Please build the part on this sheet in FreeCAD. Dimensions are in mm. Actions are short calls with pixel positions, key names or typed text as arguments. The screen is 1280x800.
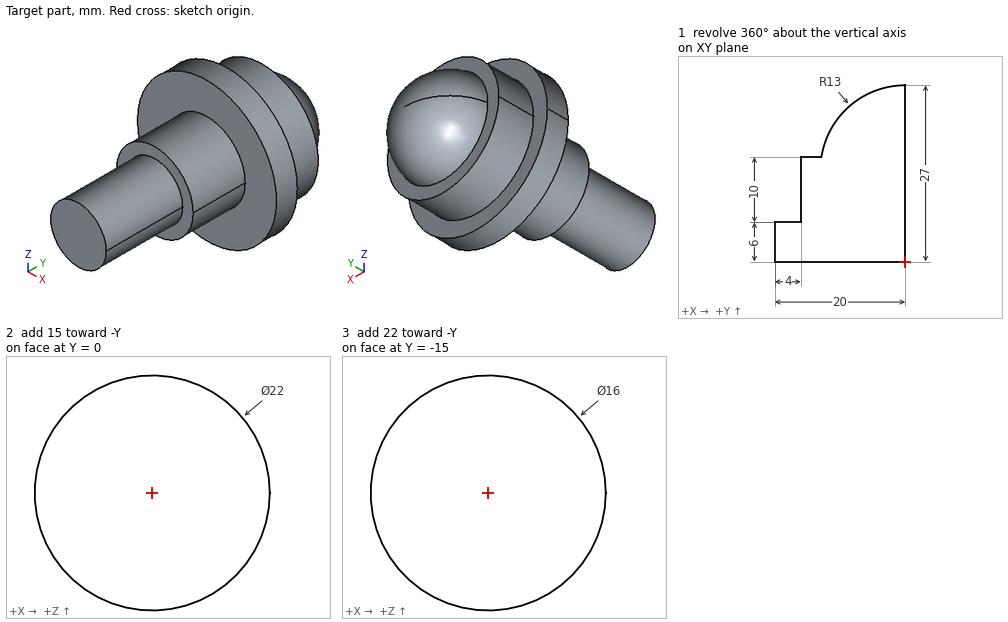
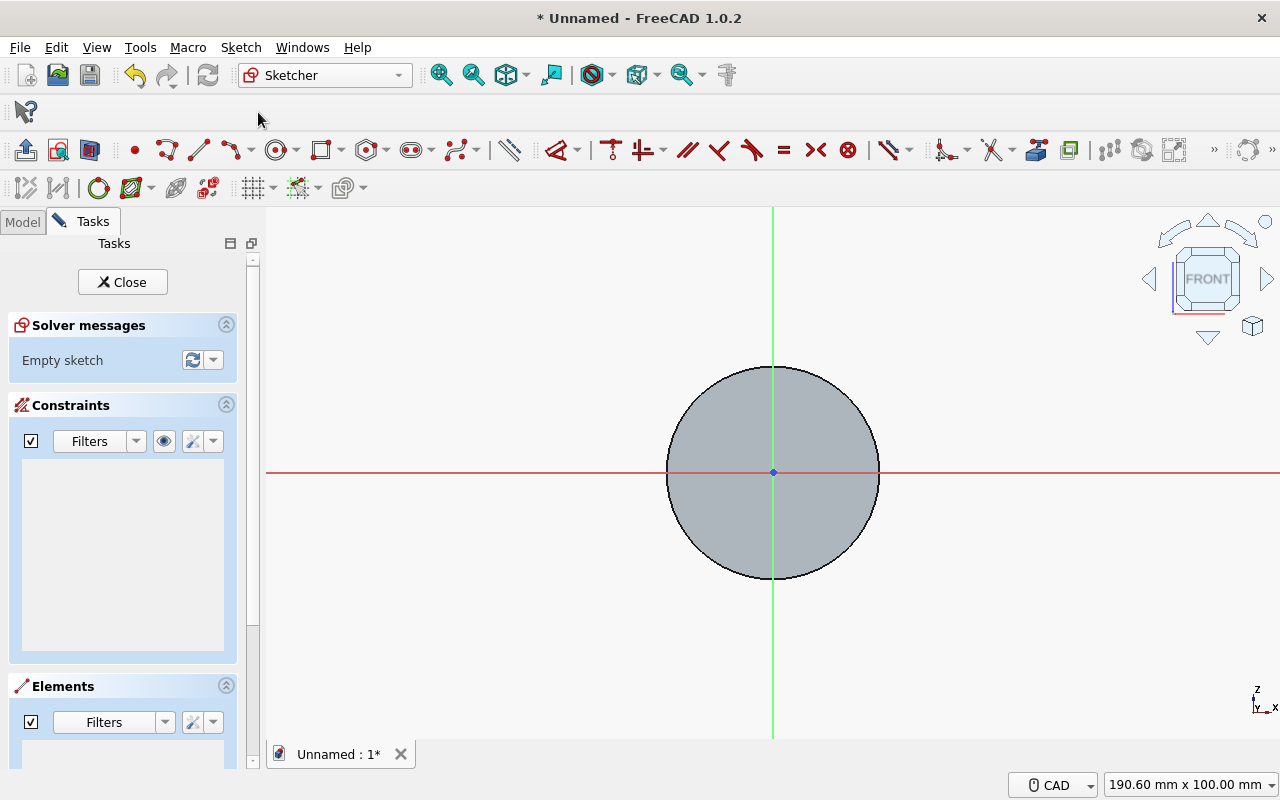
scroll(813, 473, up, 5)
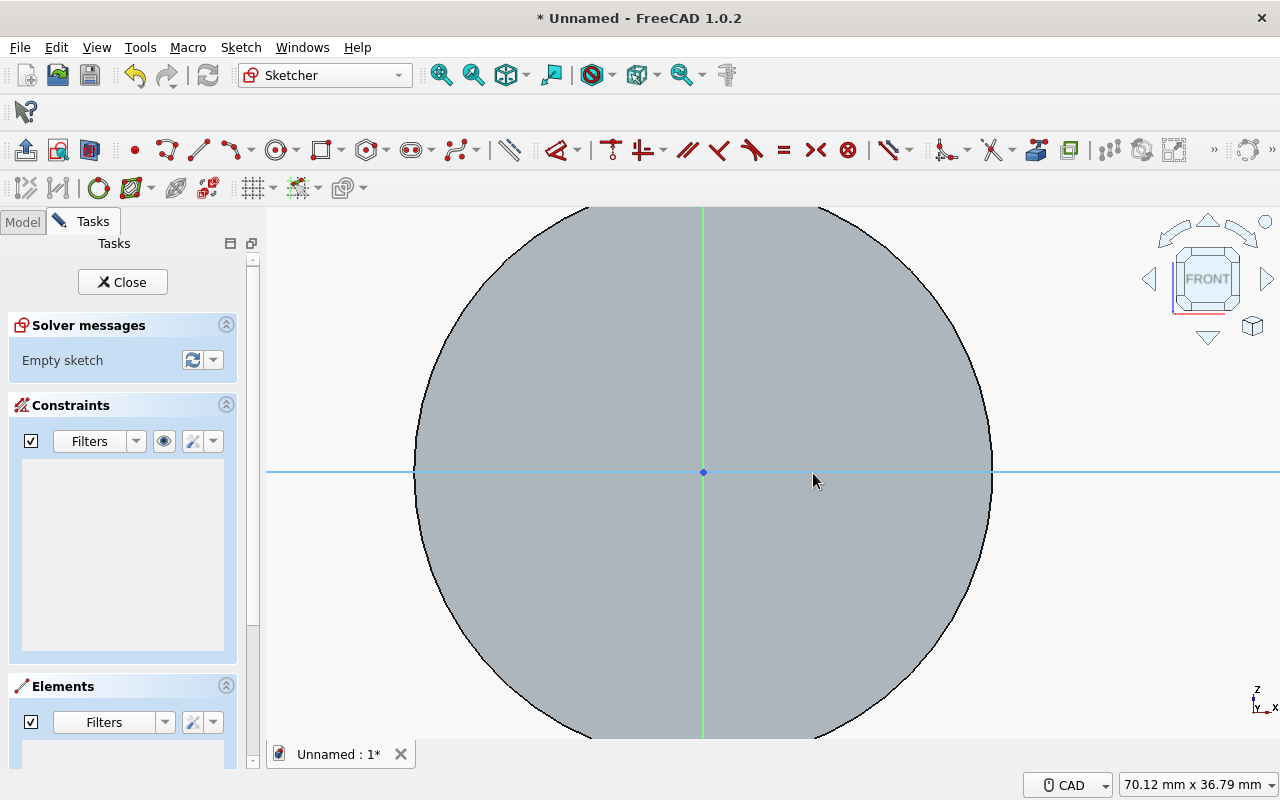
click(276, 150)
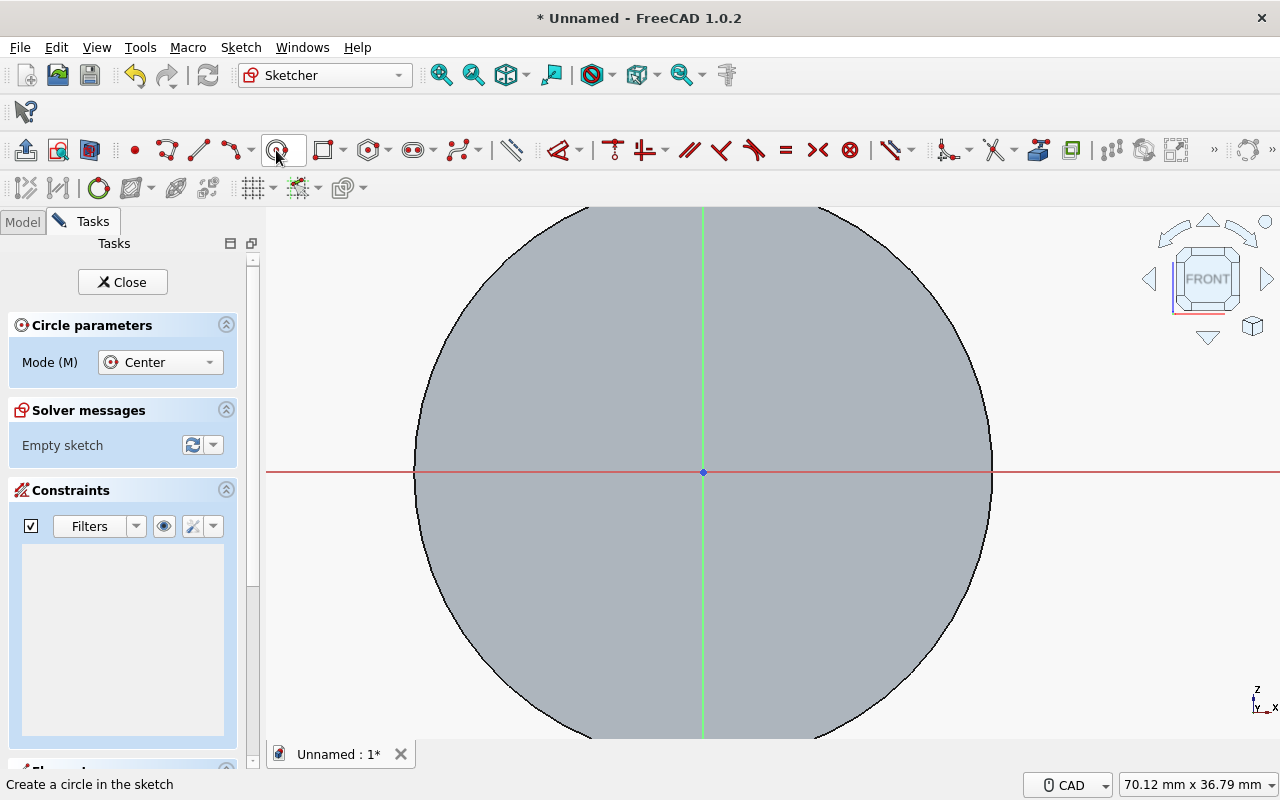
click(703, 472)
move(816, 360)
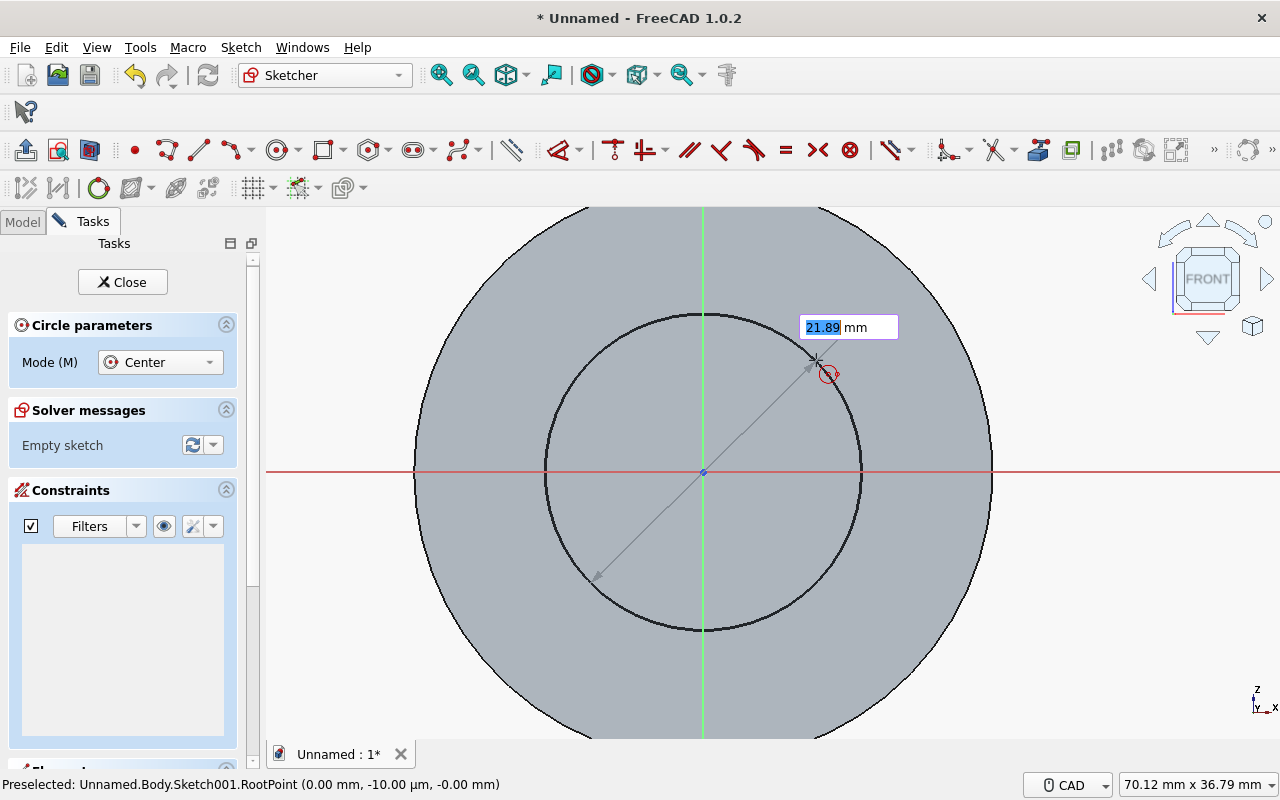
text(22)
key(Return)
key(Escape)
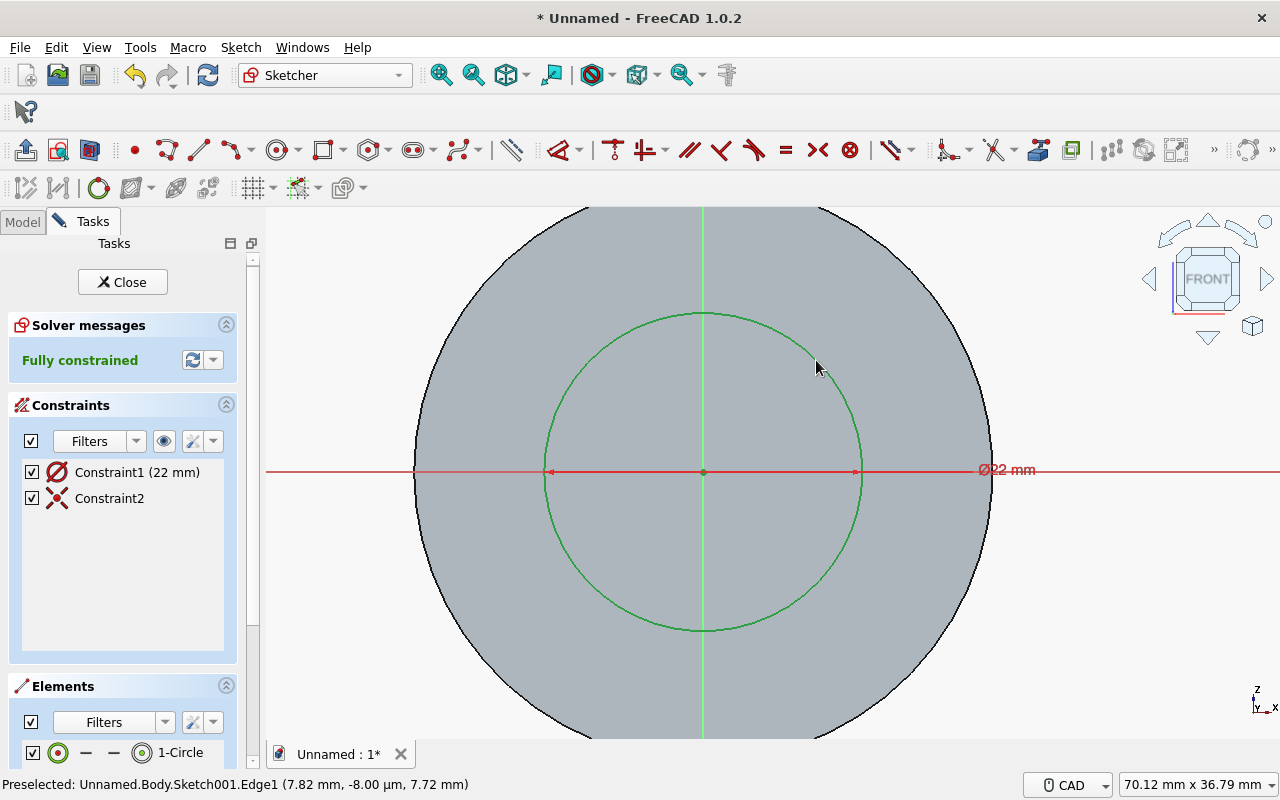
click(123, 282)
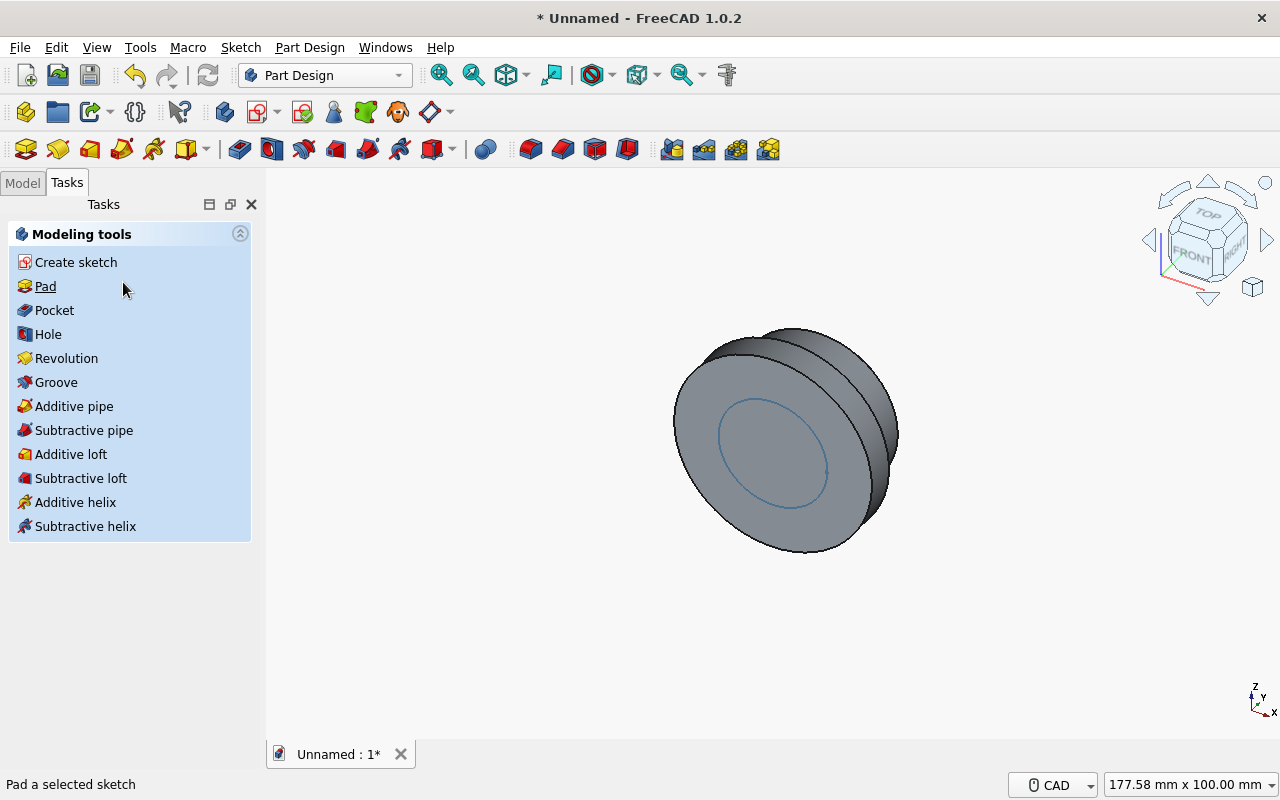
click(26, 150)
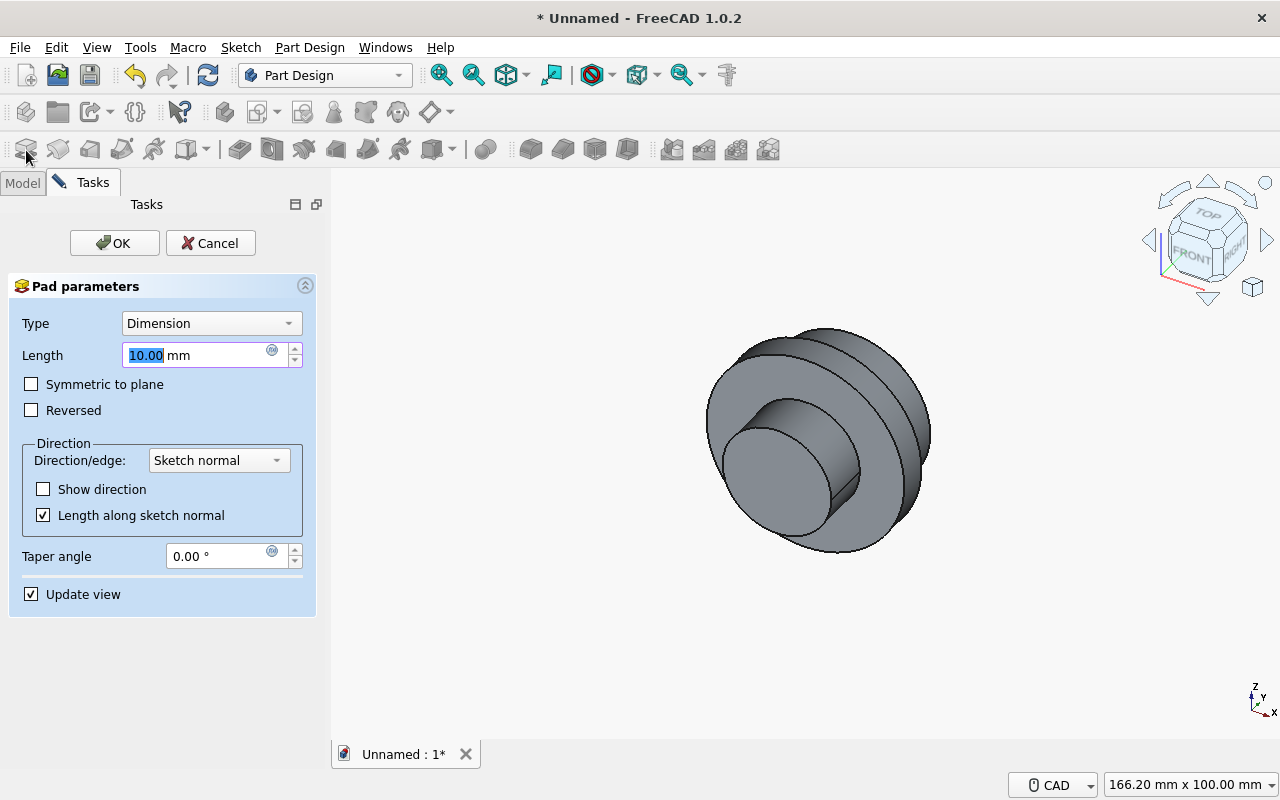
text(15)
key(Tab)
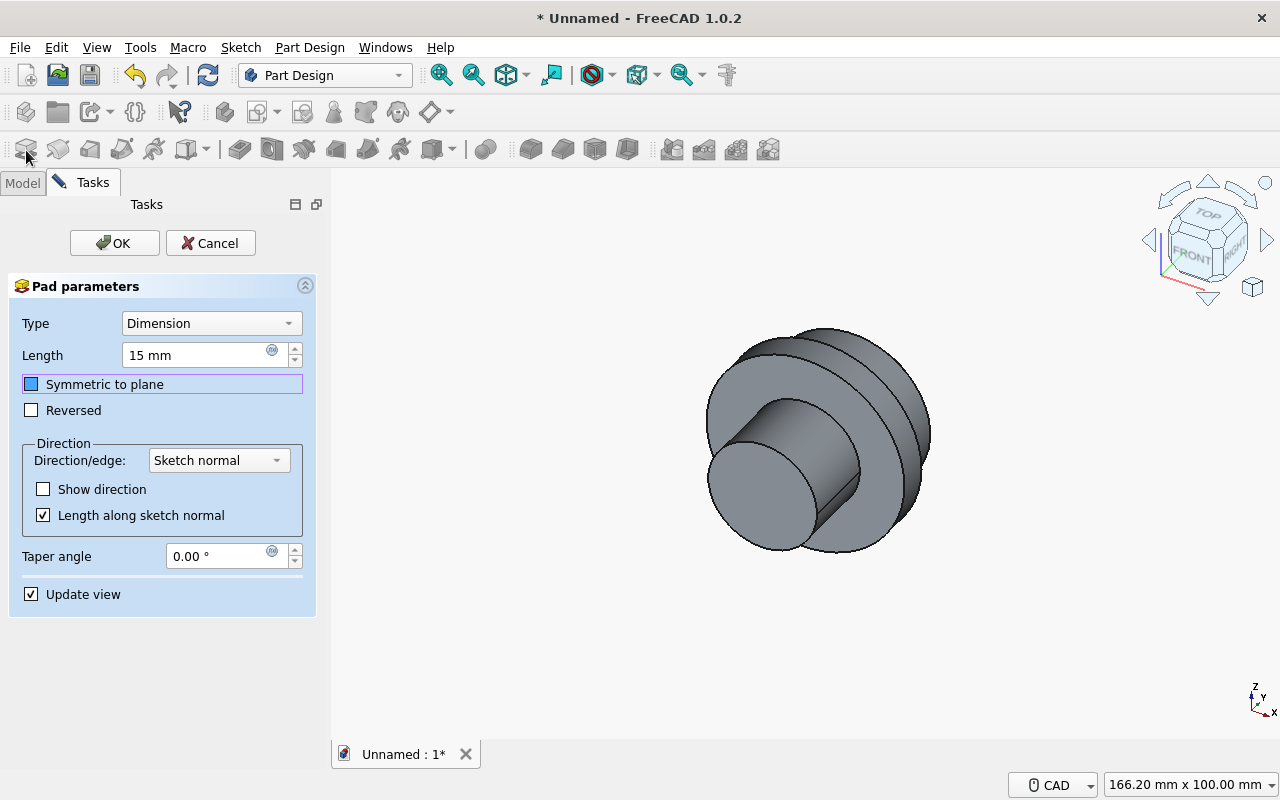
click(115, 243)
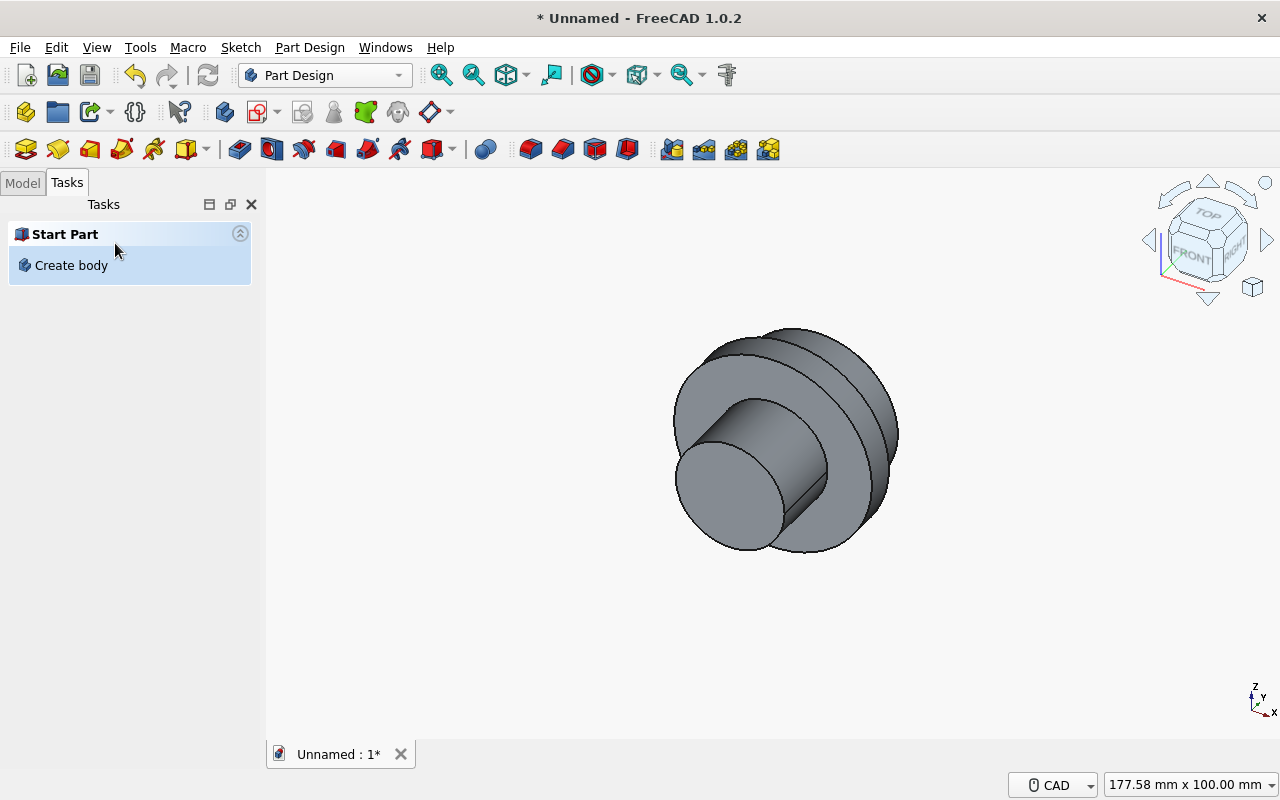
click(730, 495)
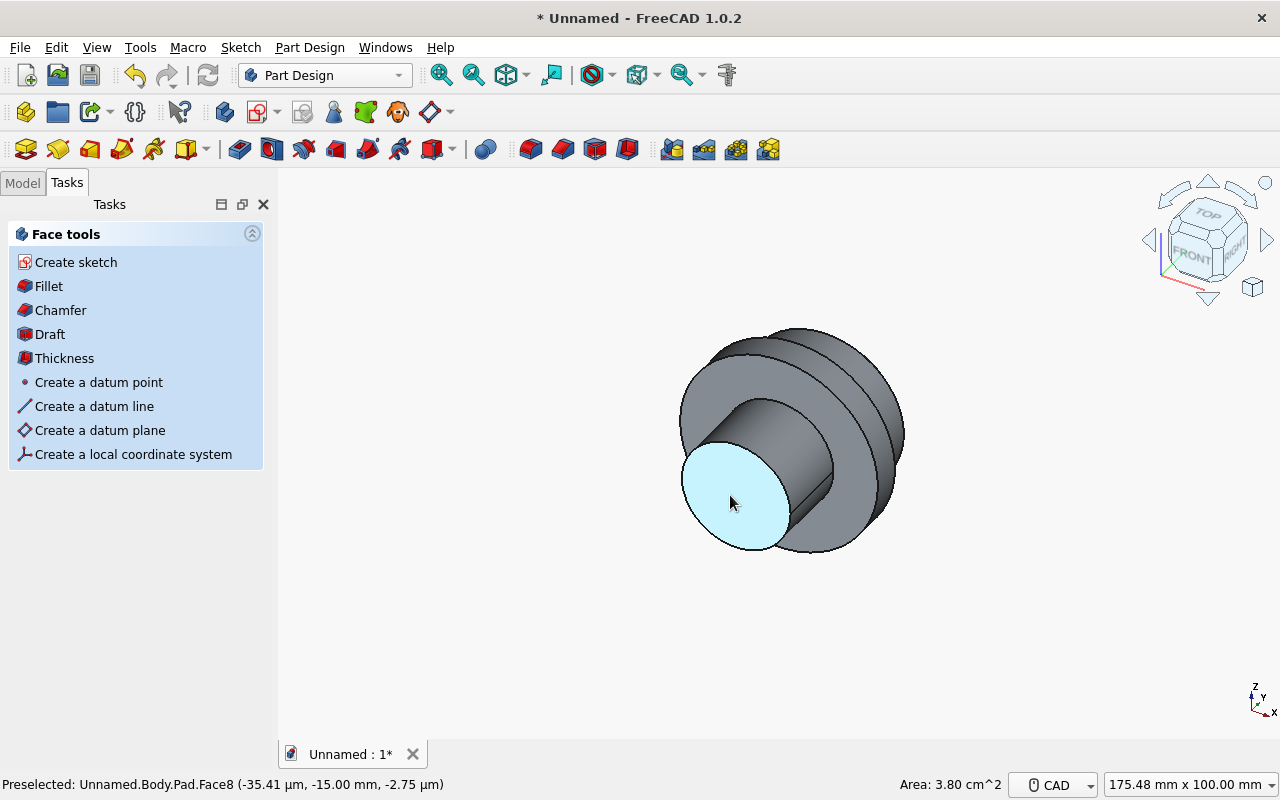
click(258, 112)